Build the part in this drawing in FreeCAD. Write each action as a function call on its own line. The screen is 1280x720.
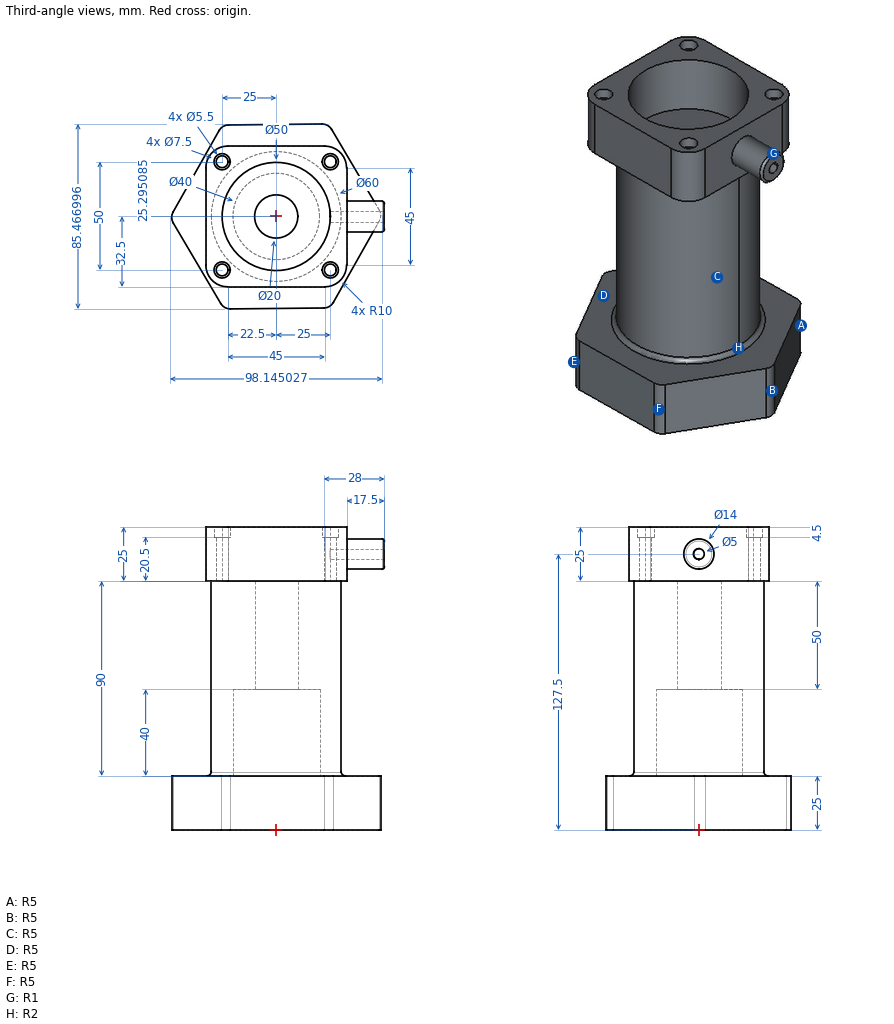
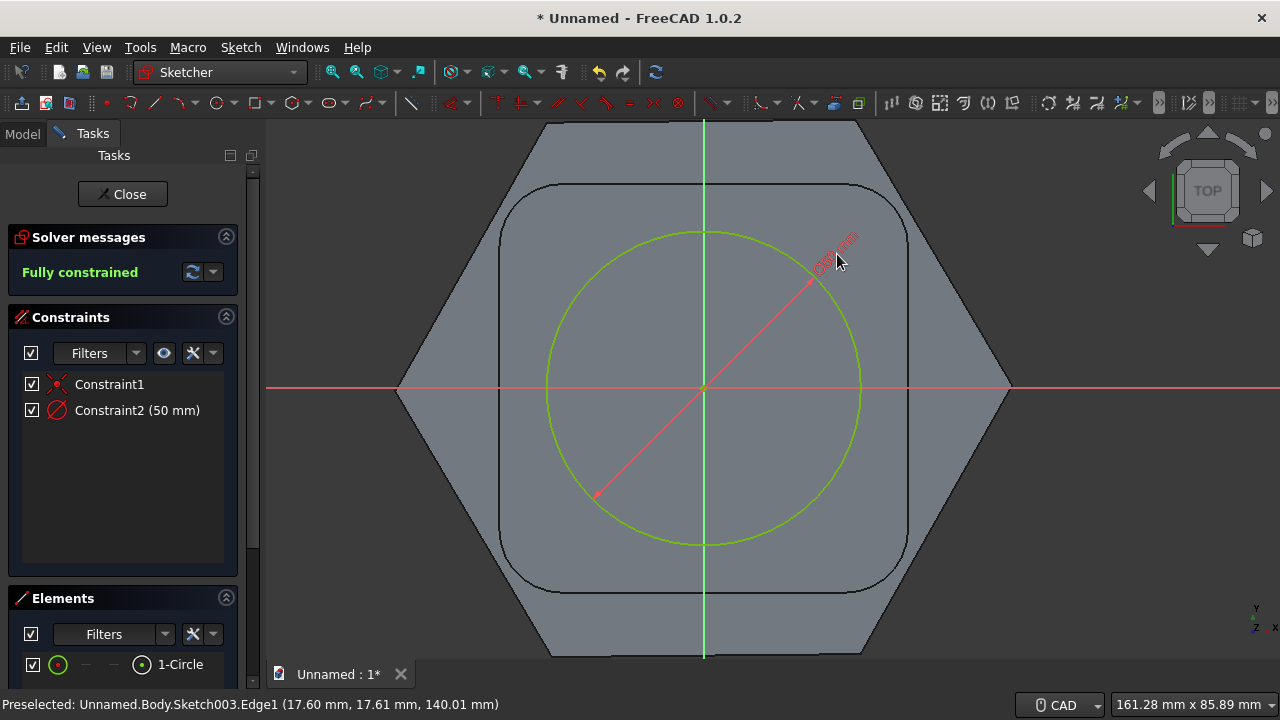
click(123, 194)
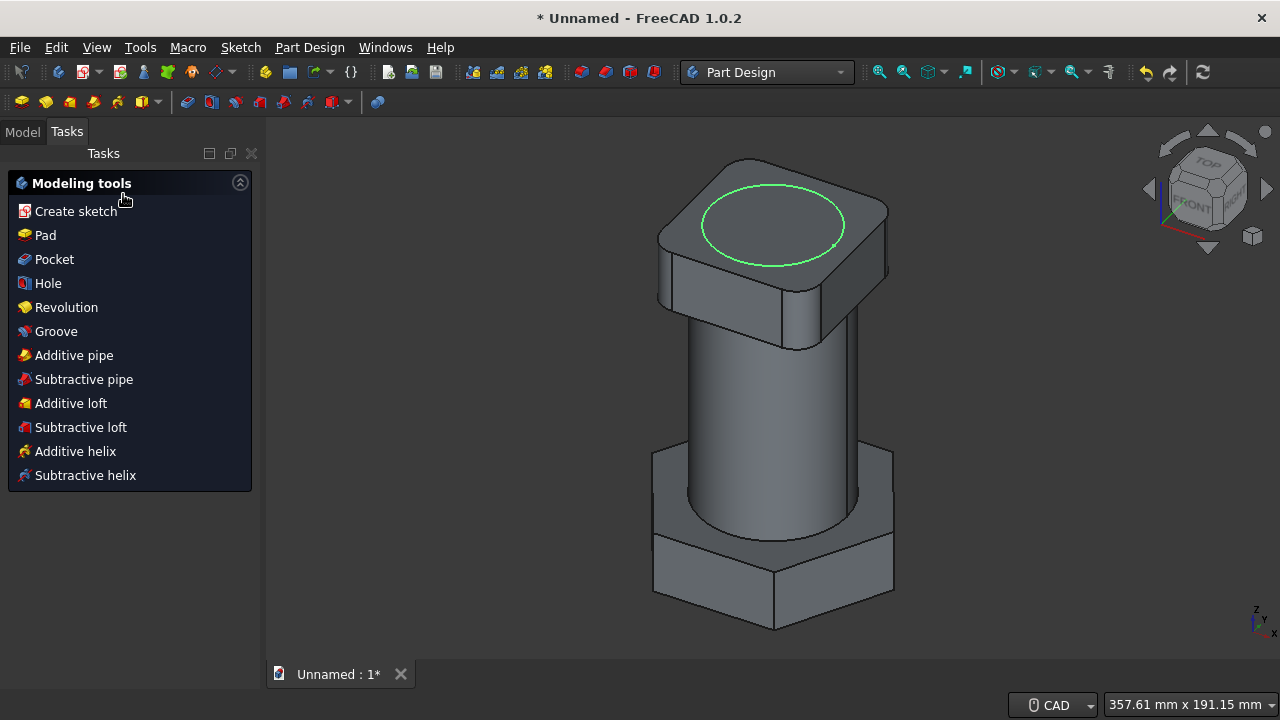
click(188, 102)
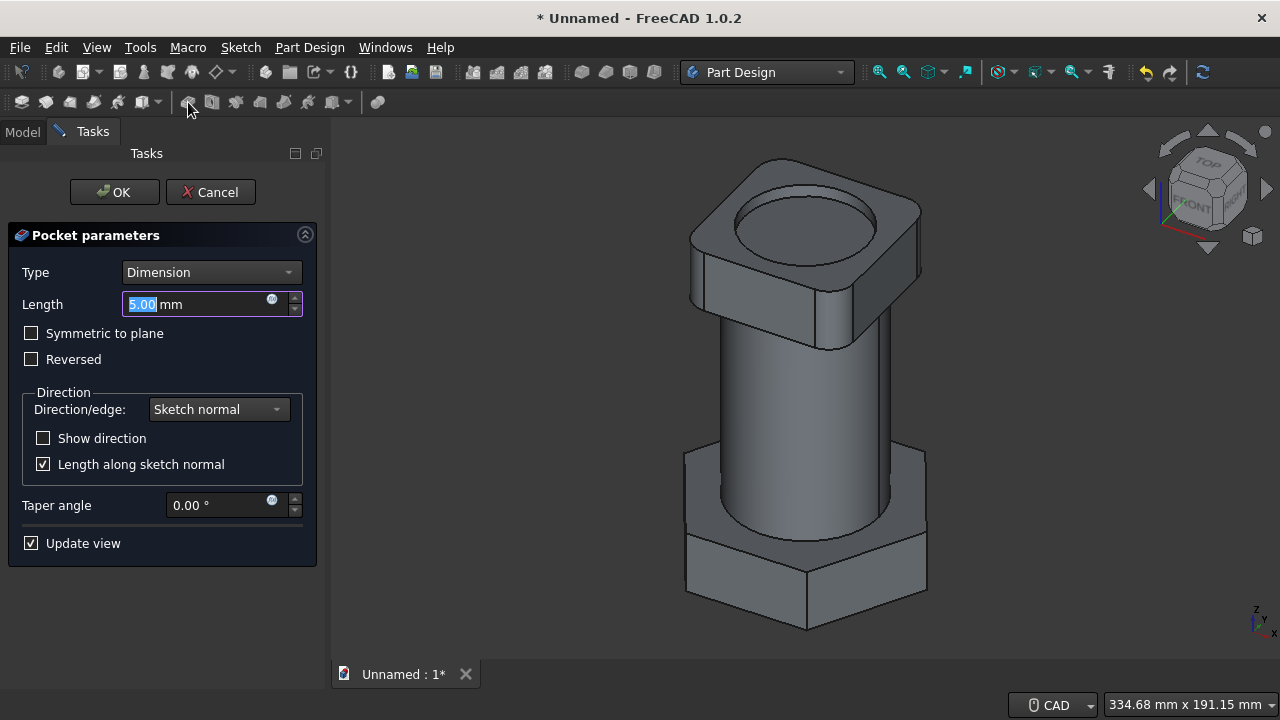
text(25)
key(Tab)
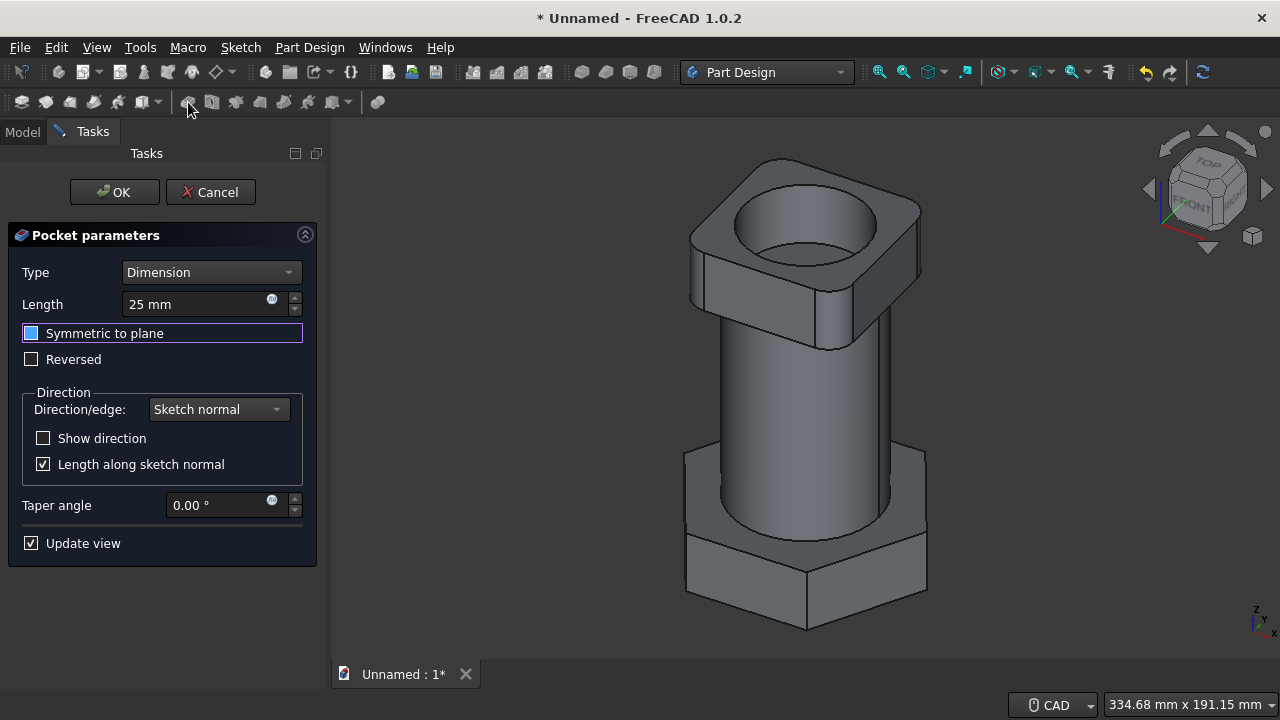
click(115, 192)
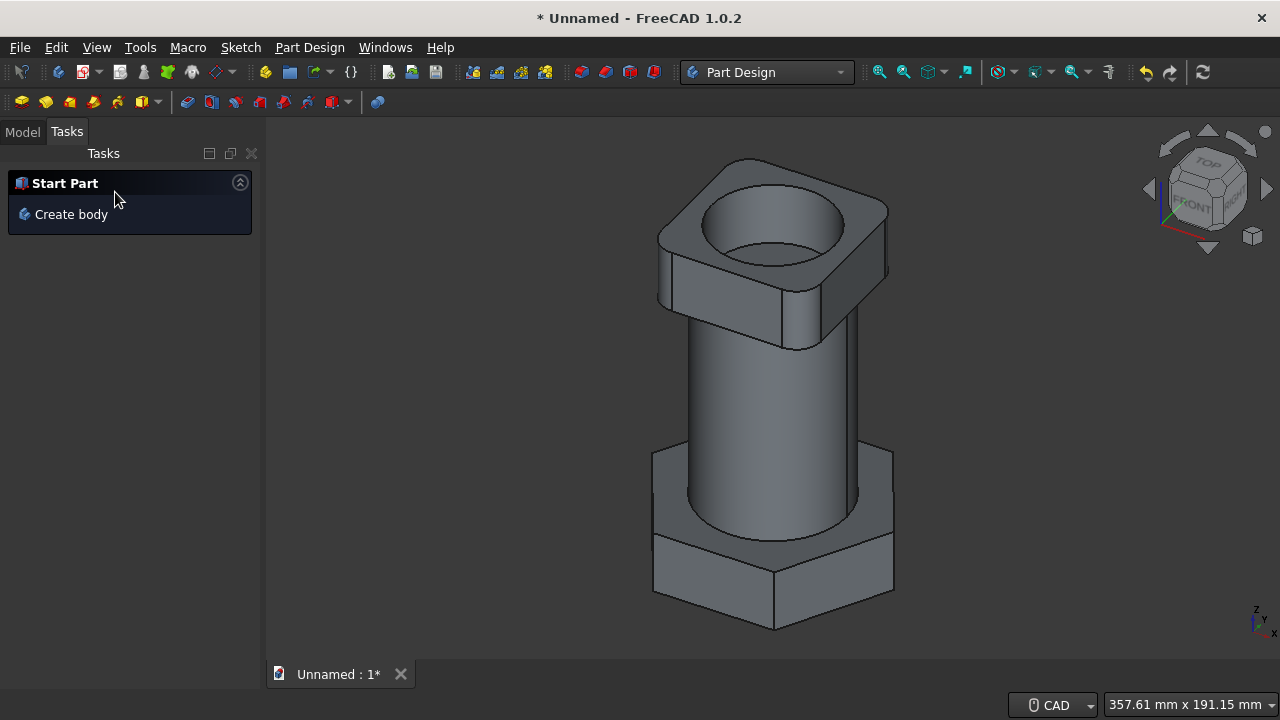
key(0)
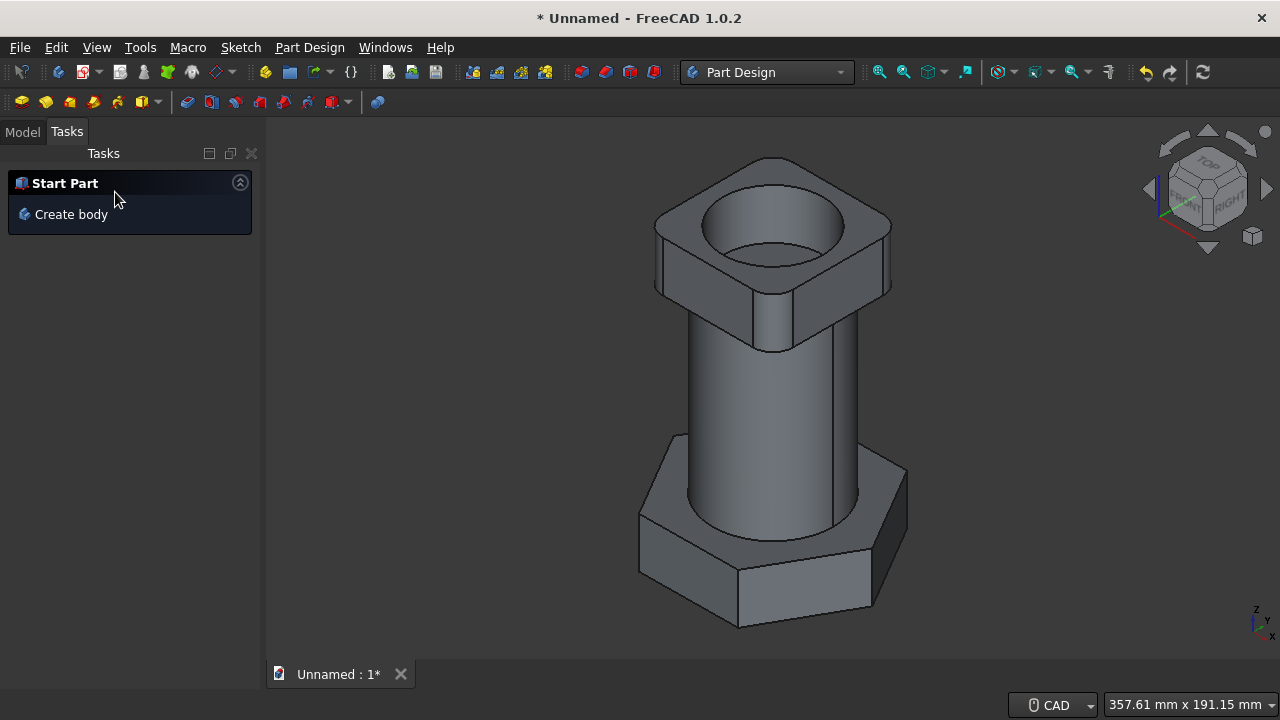
key(2)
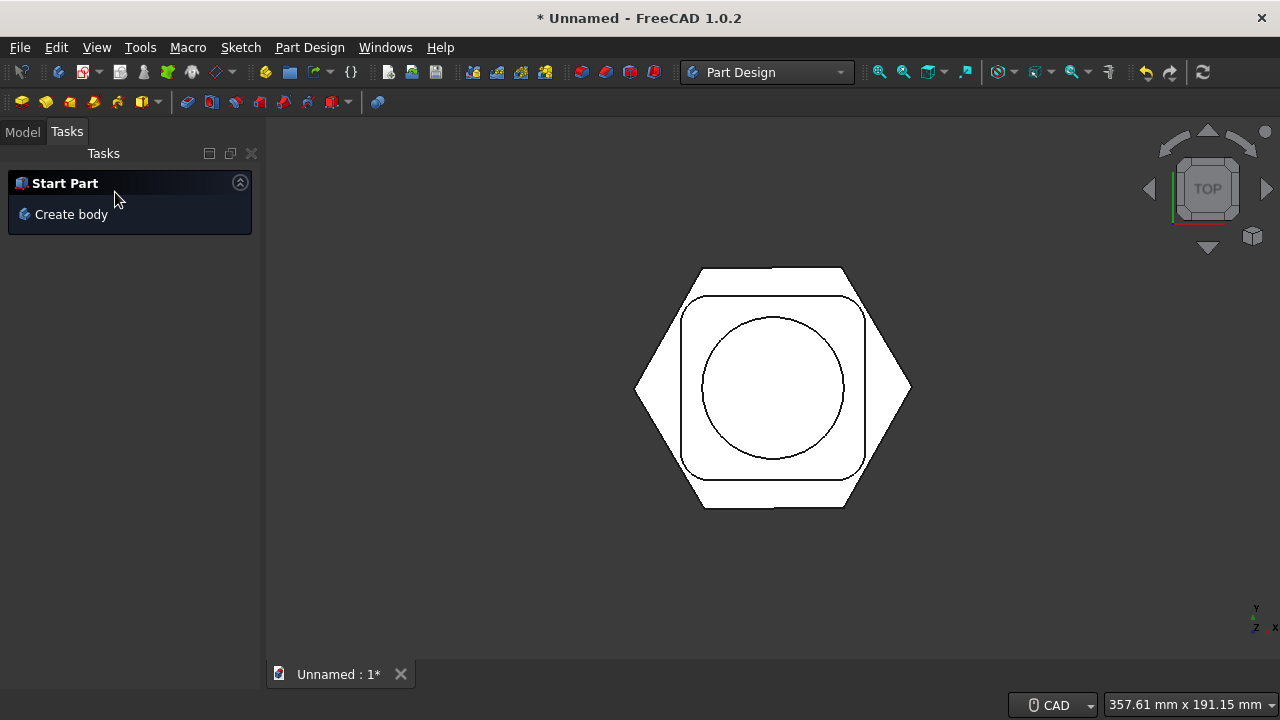
click(880, 72)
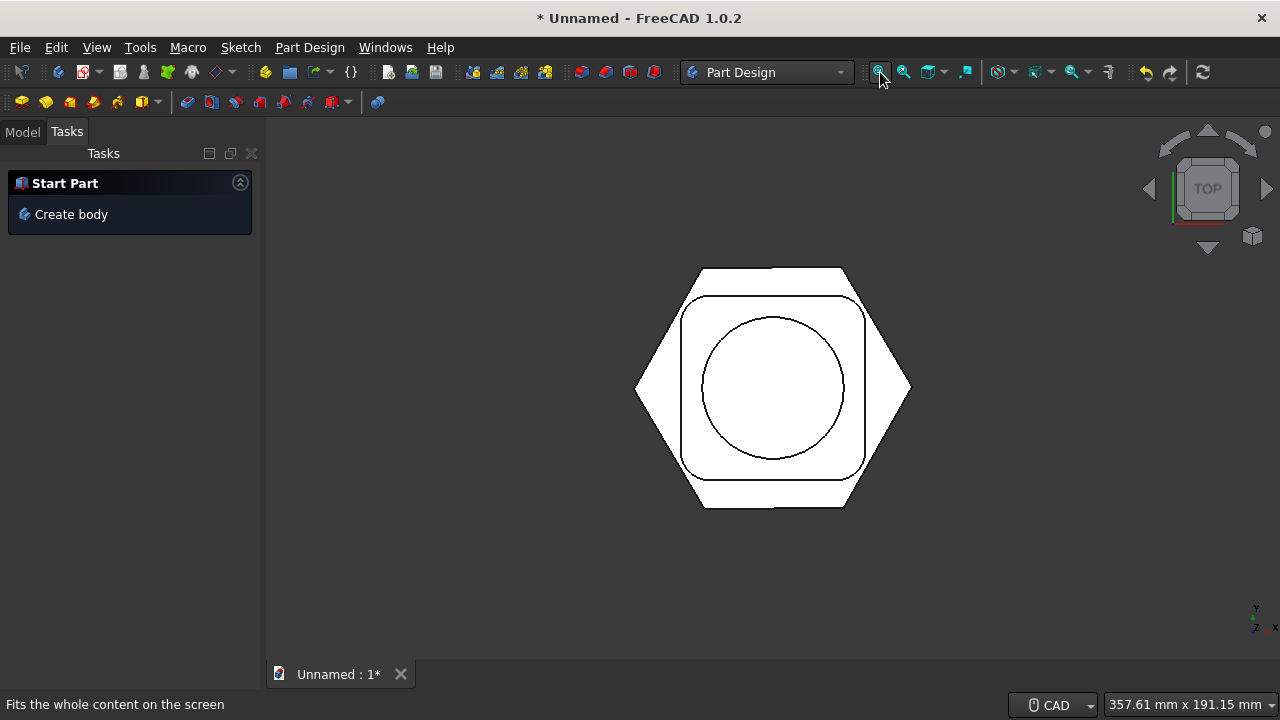
click(773, 387)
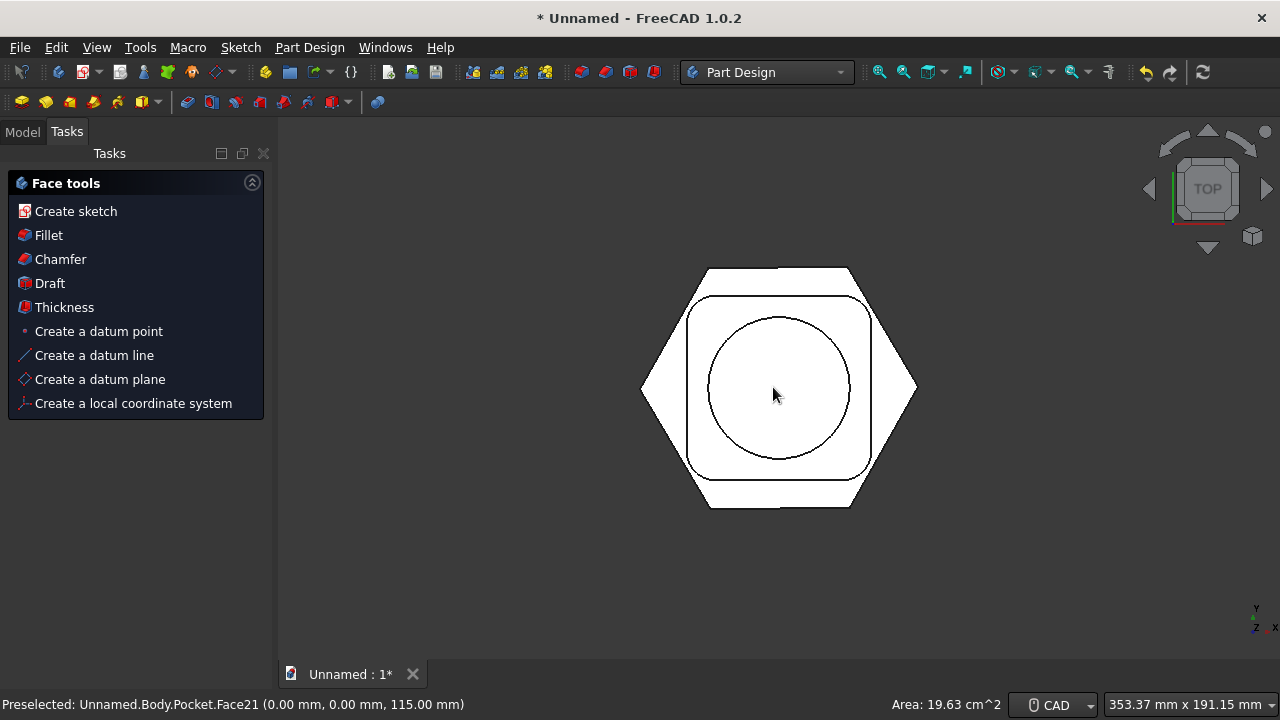
click(84, 72)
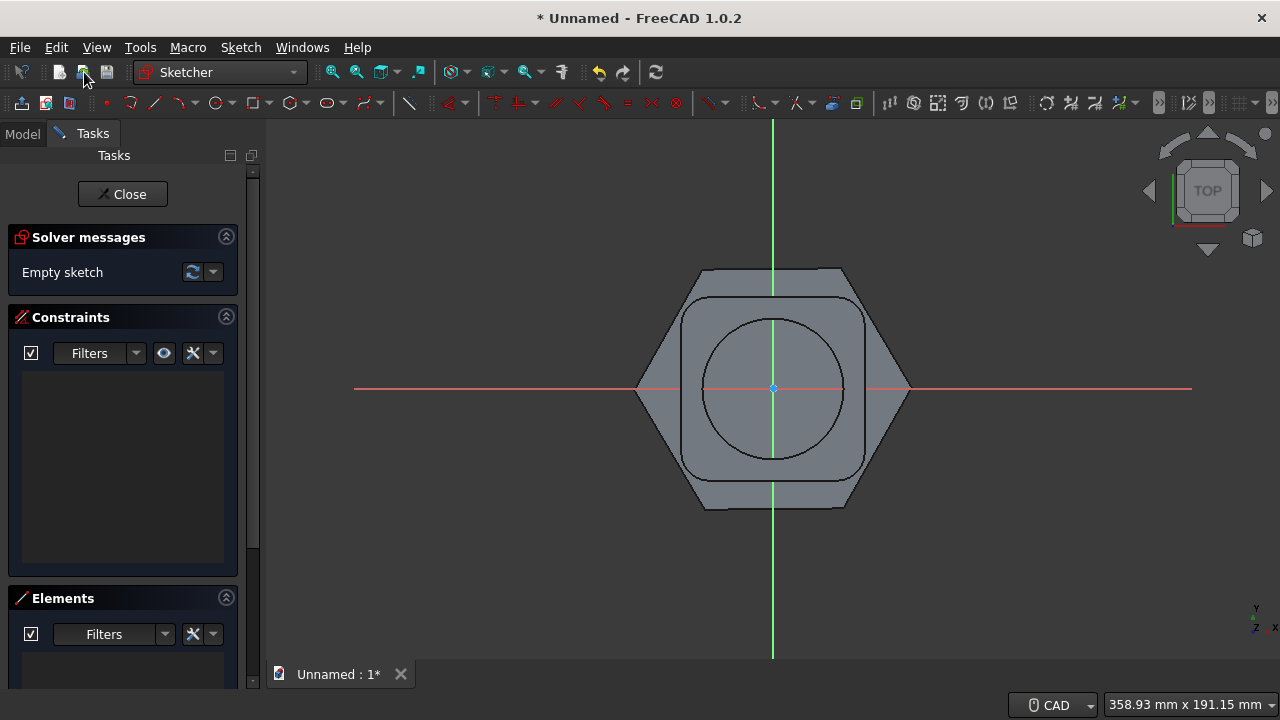
click(70, 104)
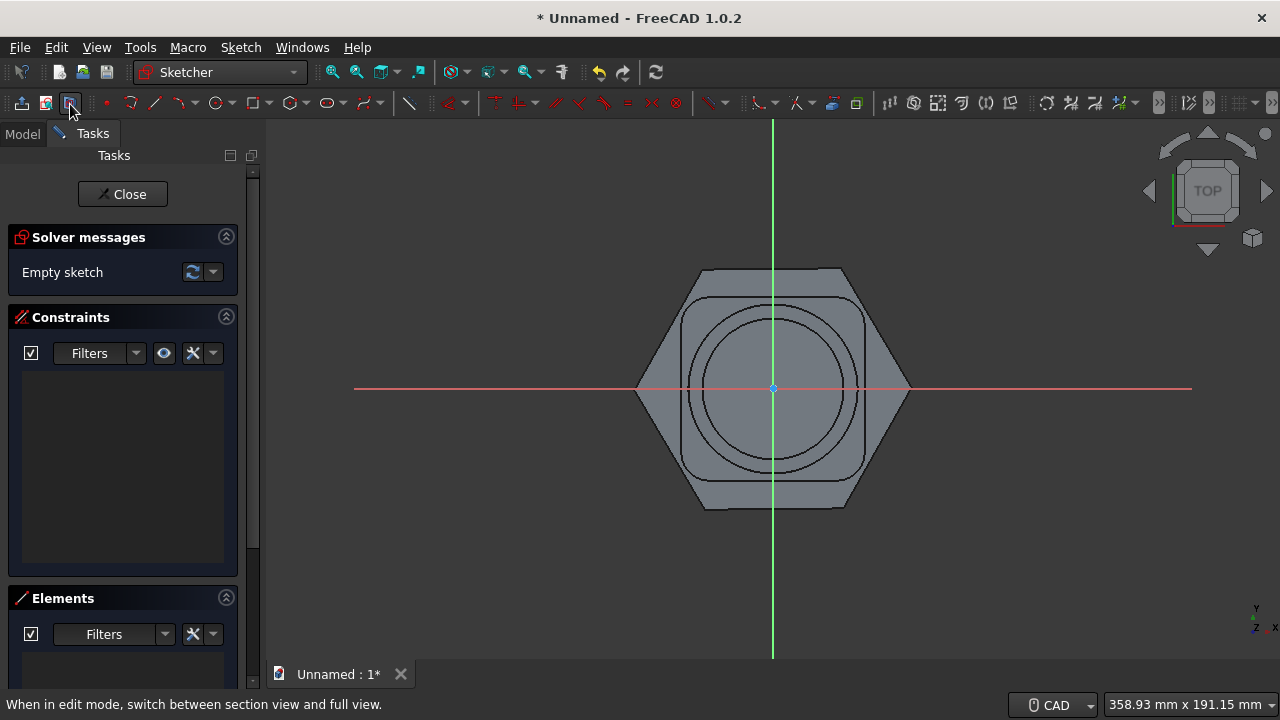
scroll(787, 389, up, 9)